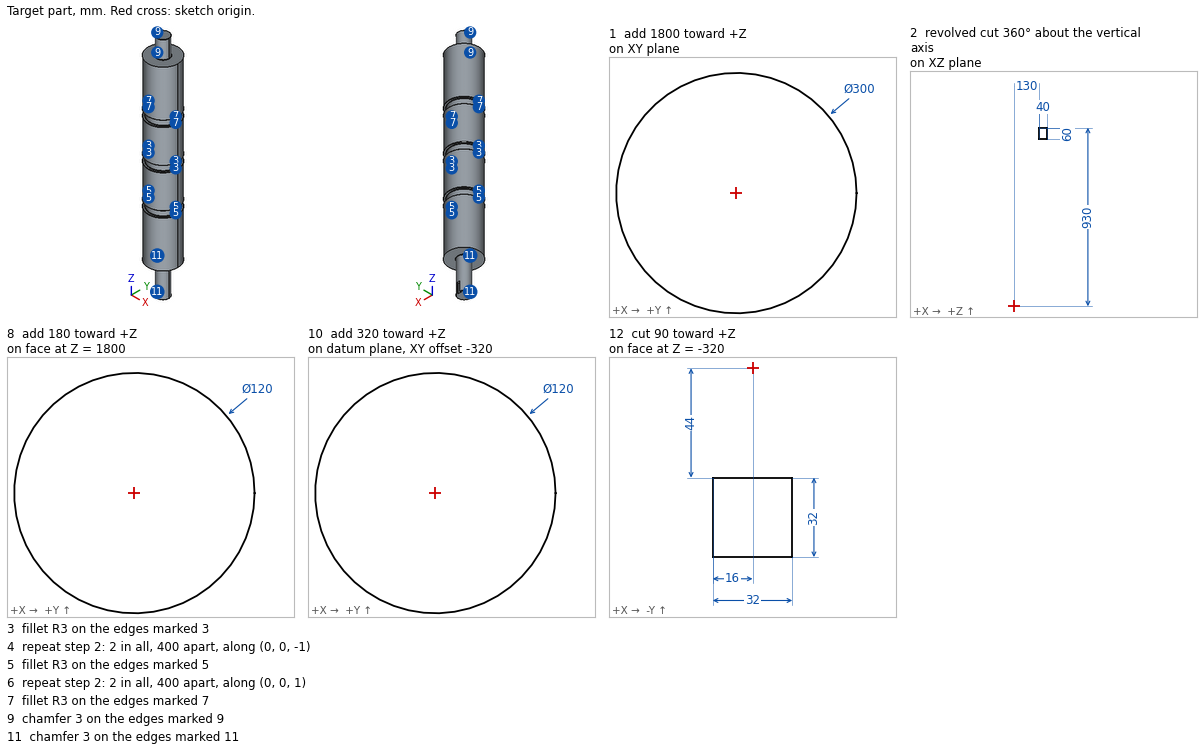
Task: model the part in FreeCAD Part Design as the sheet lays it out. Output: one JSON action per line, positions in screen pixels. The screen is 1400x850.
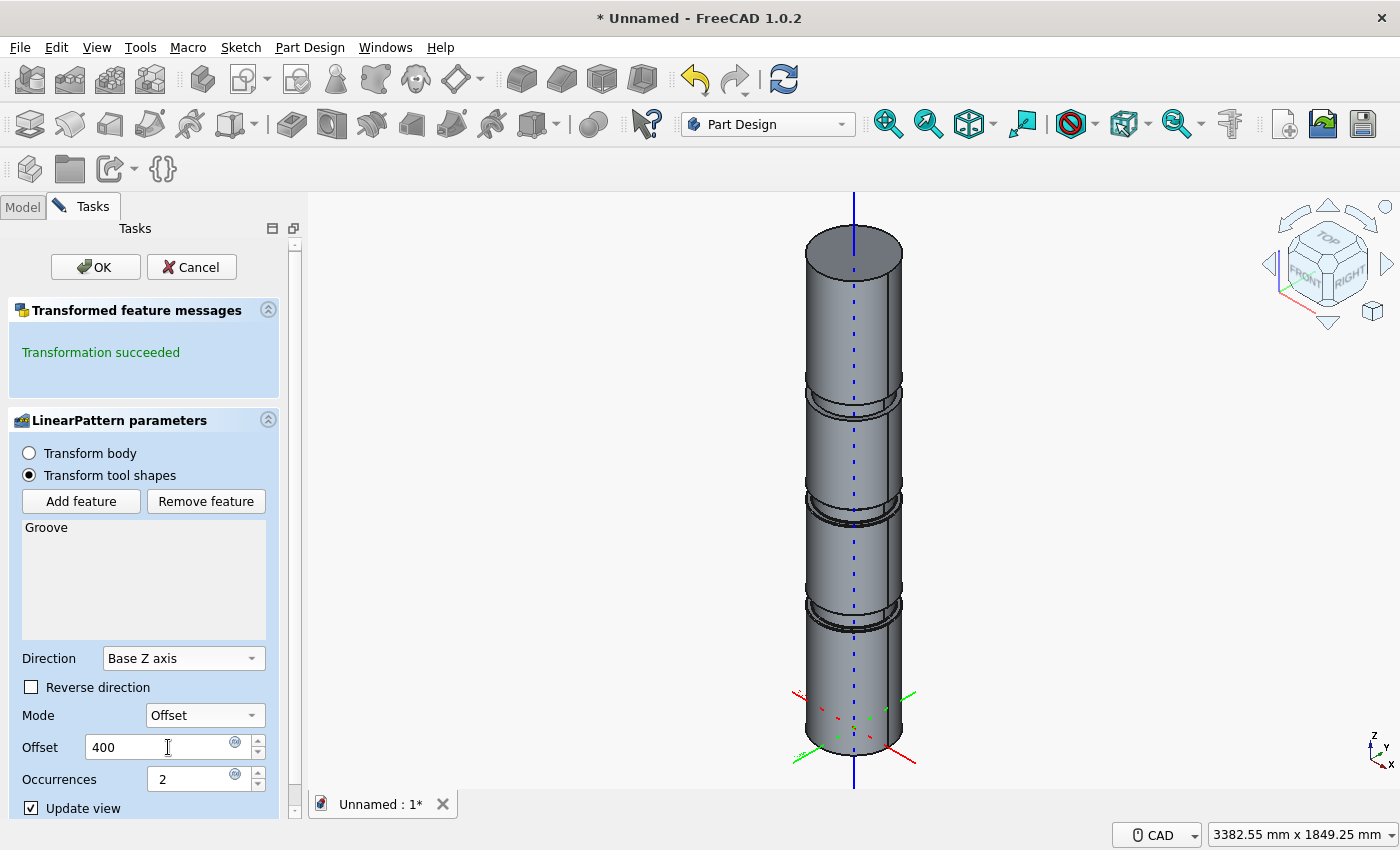
{"action": "triple_click", "coordinate": [198, 779]}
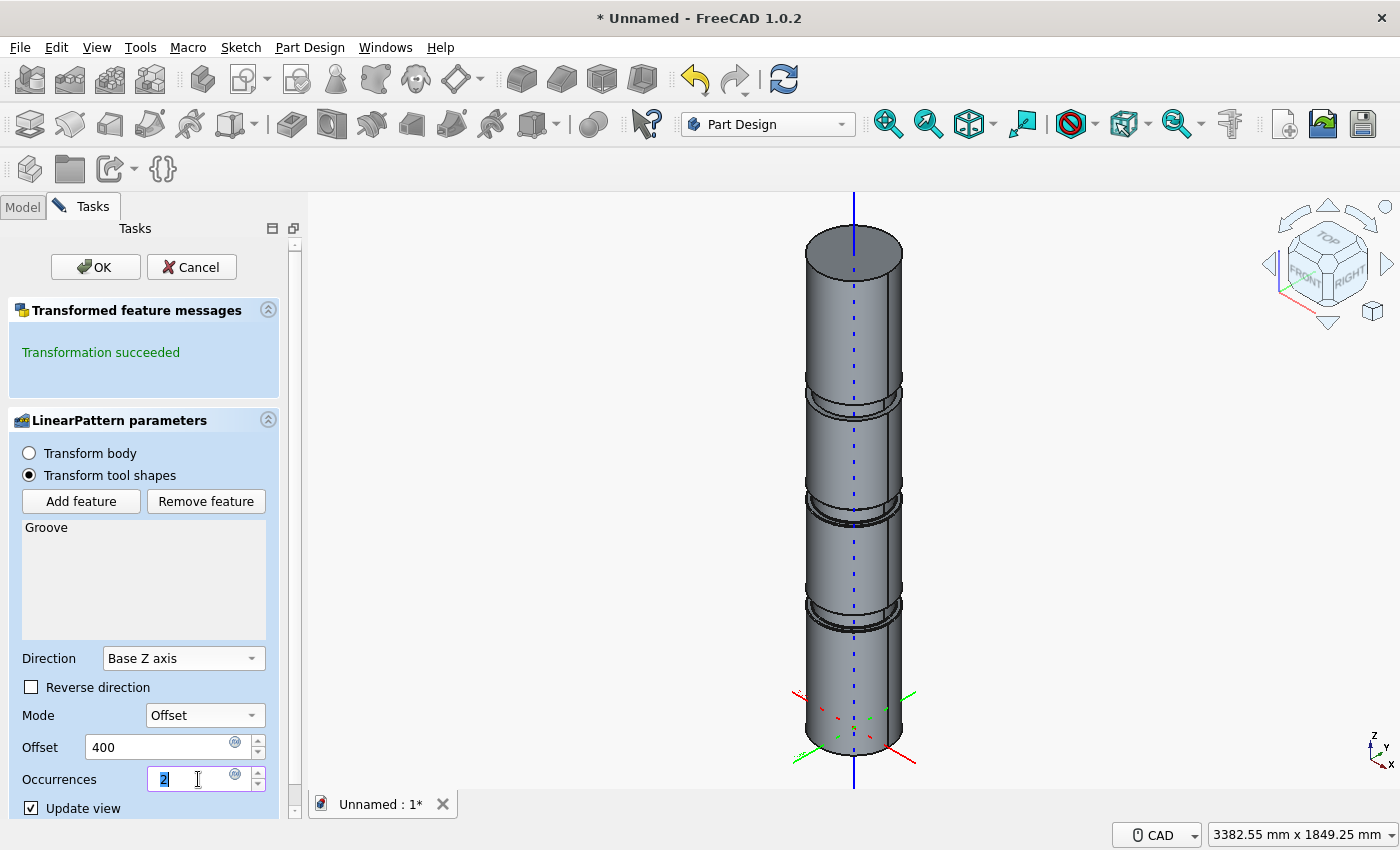
{"action": "type", "text": "2"}
{"action": "key", "text": "Tab"}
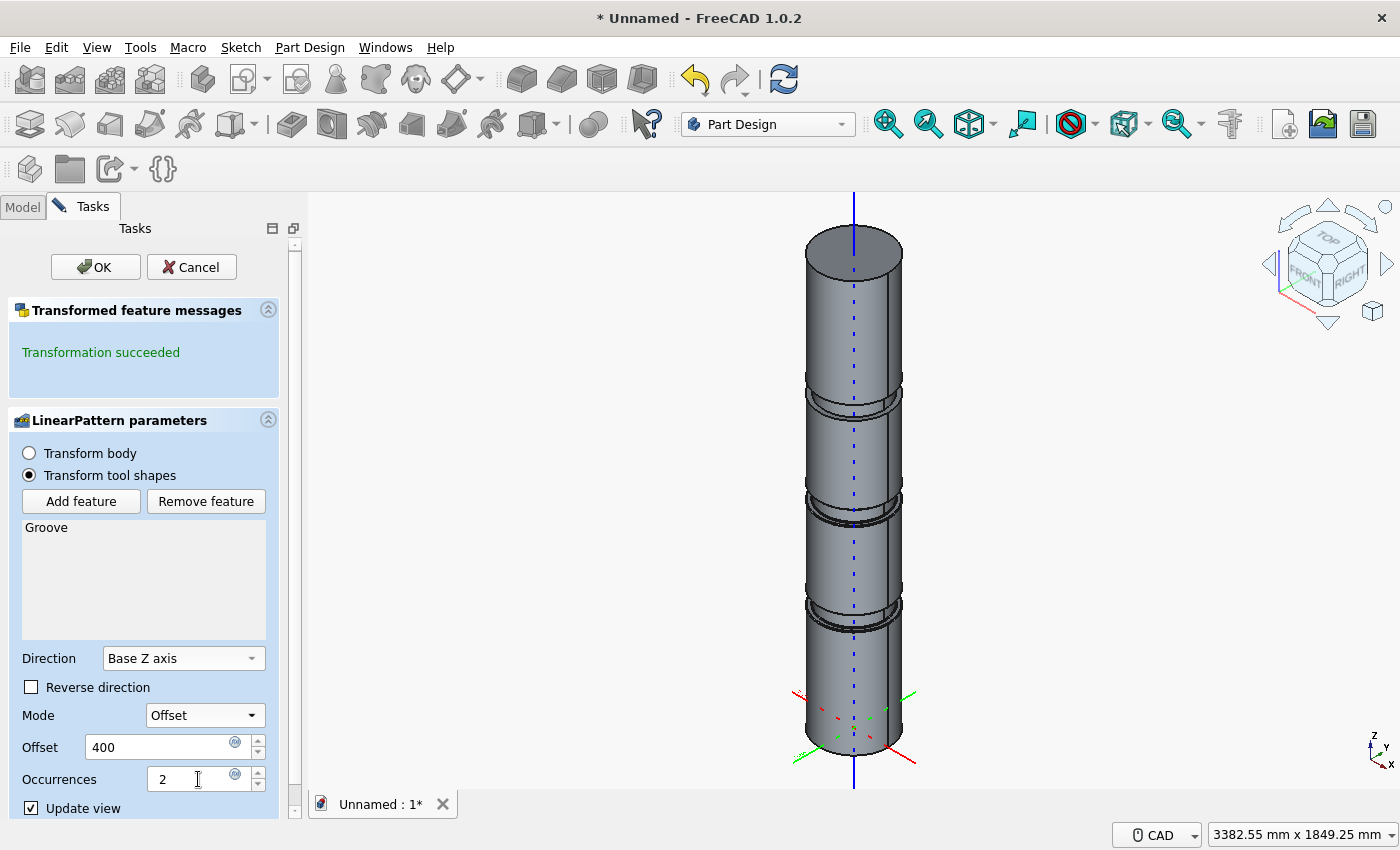
{"action": "left_click", "coordinate": [96, 267]}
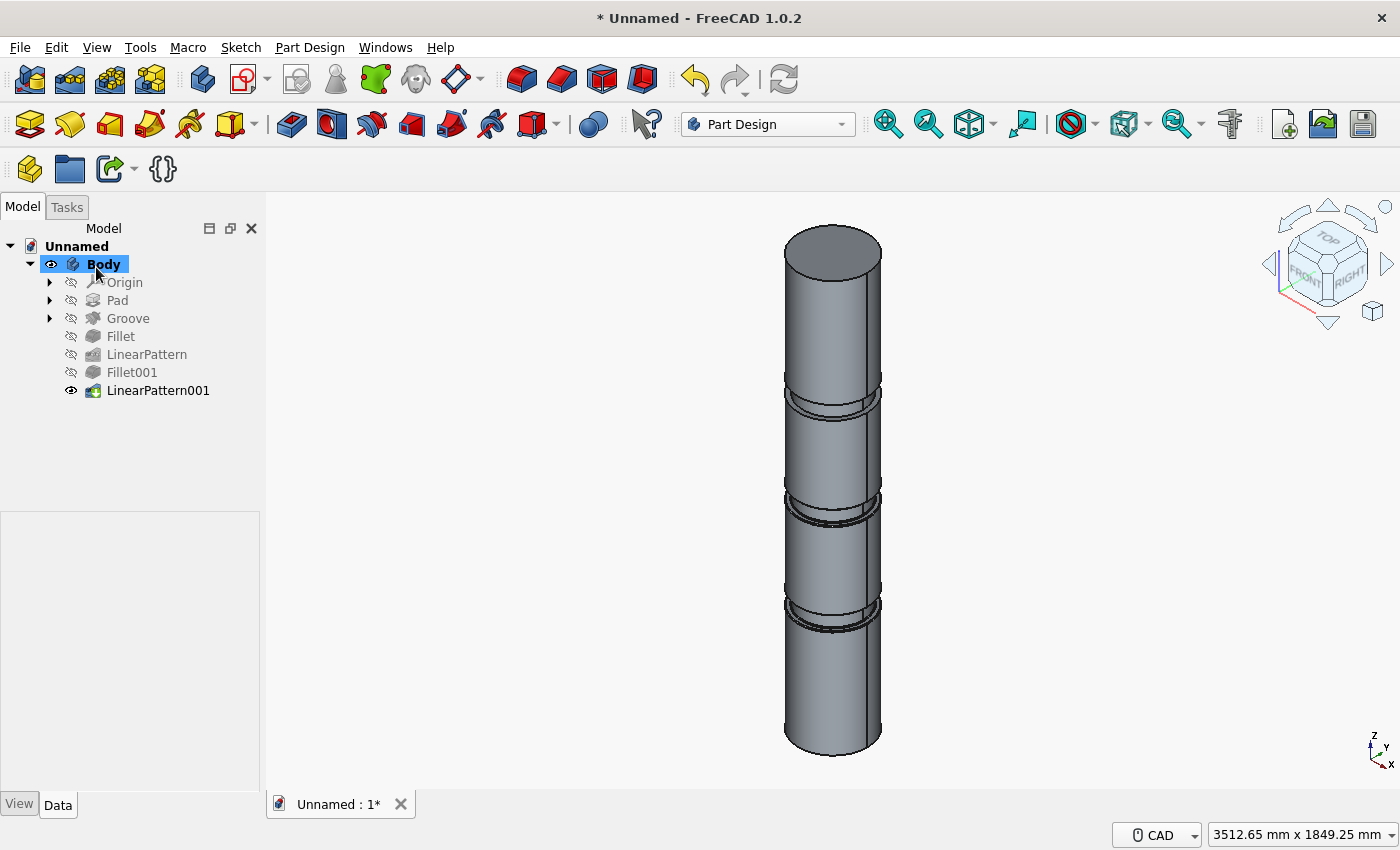
{"action": "left_click", "coordinate": [790, 405]}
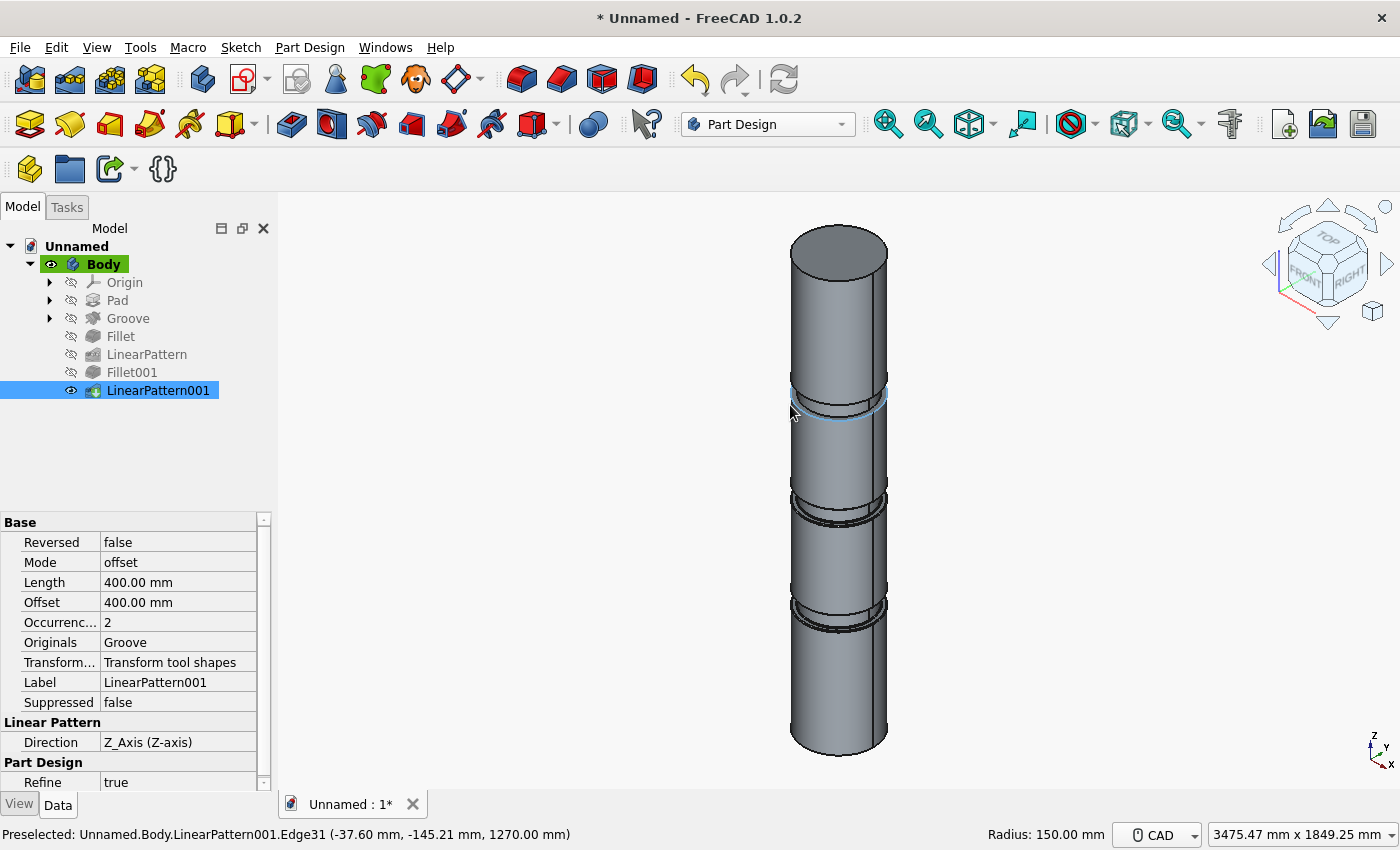
{"action": "key", "text": "2"}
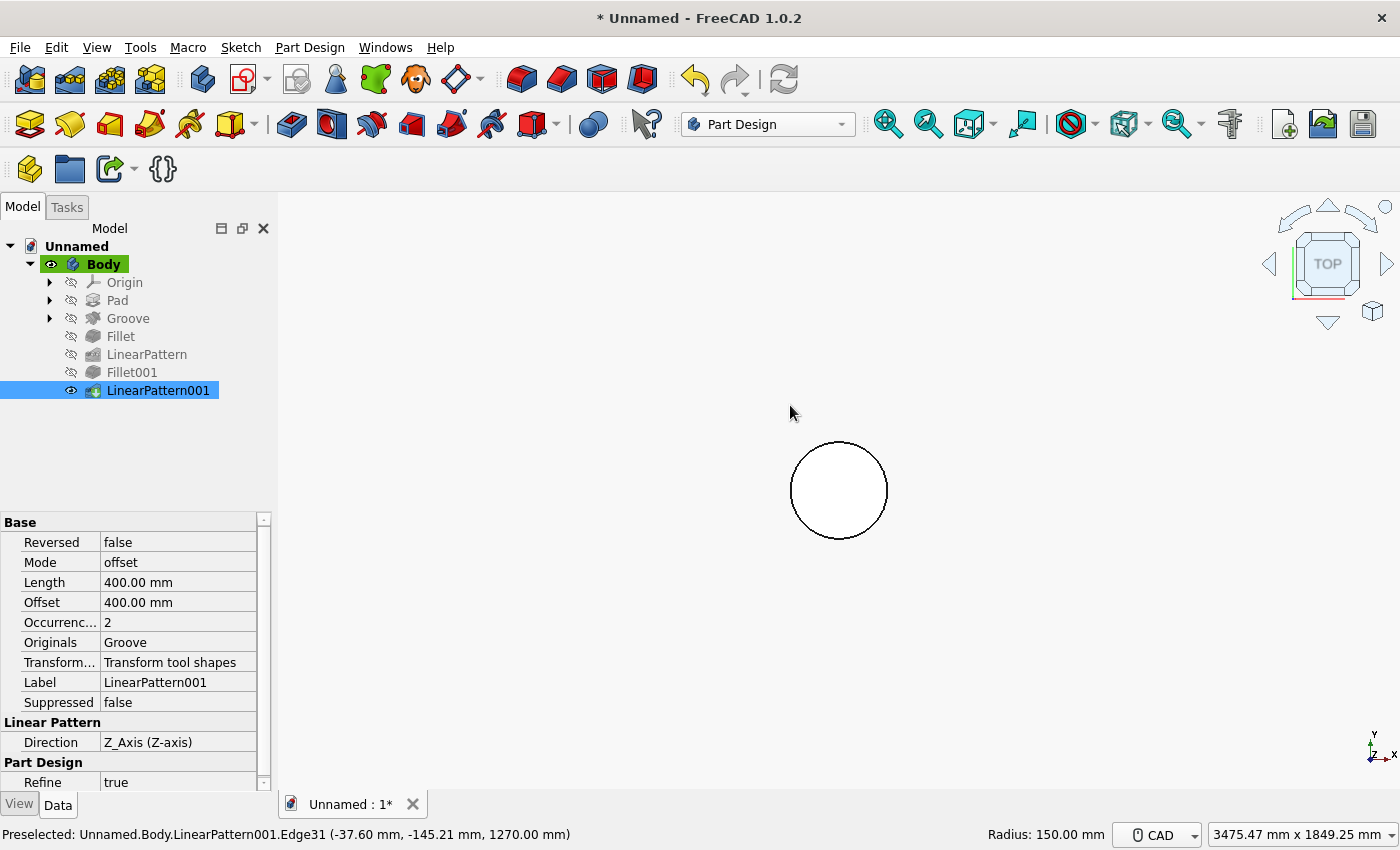
{"action": "left_click", "coordinate": [890, 124]}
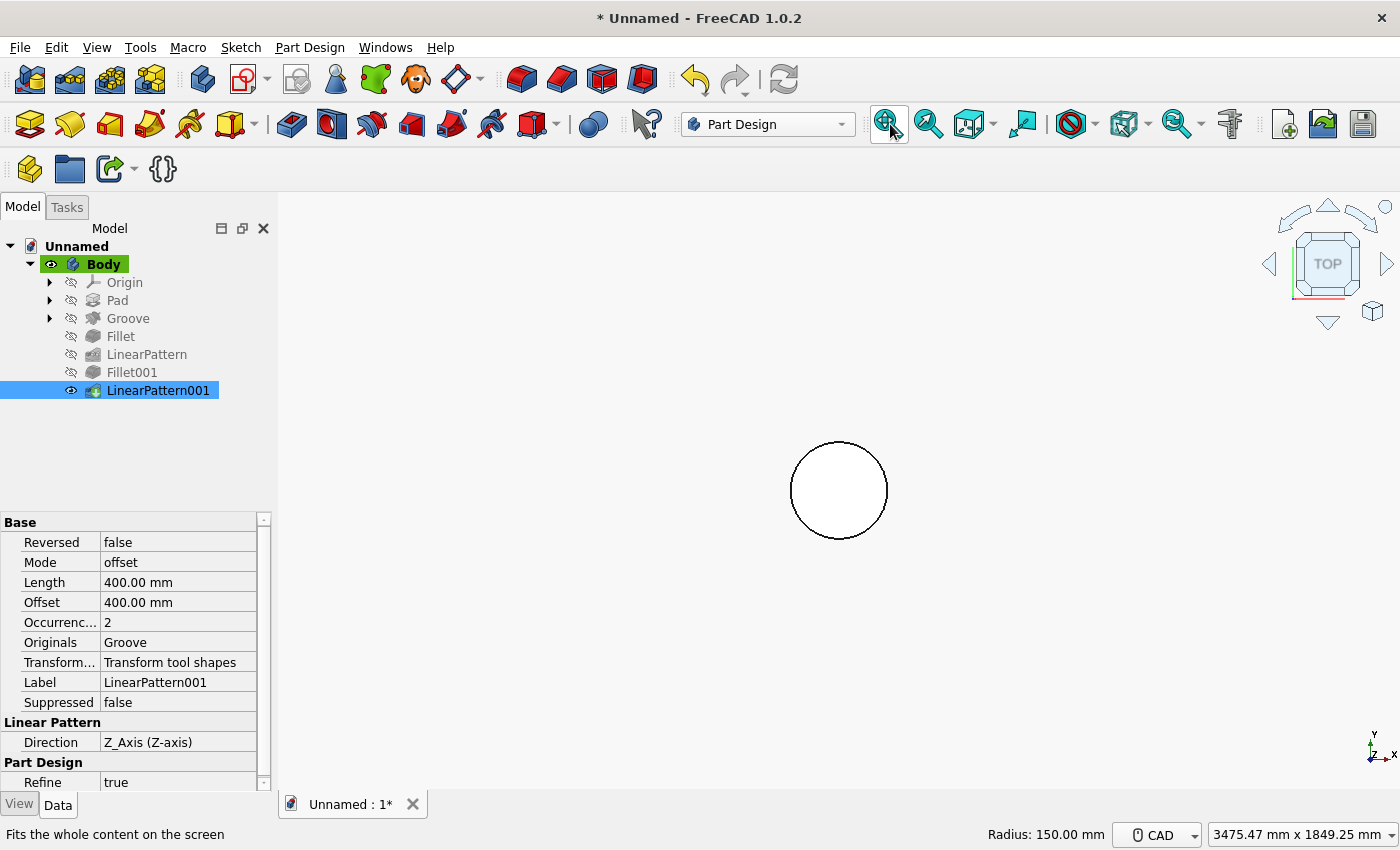
{"action": "key", "text": "0"}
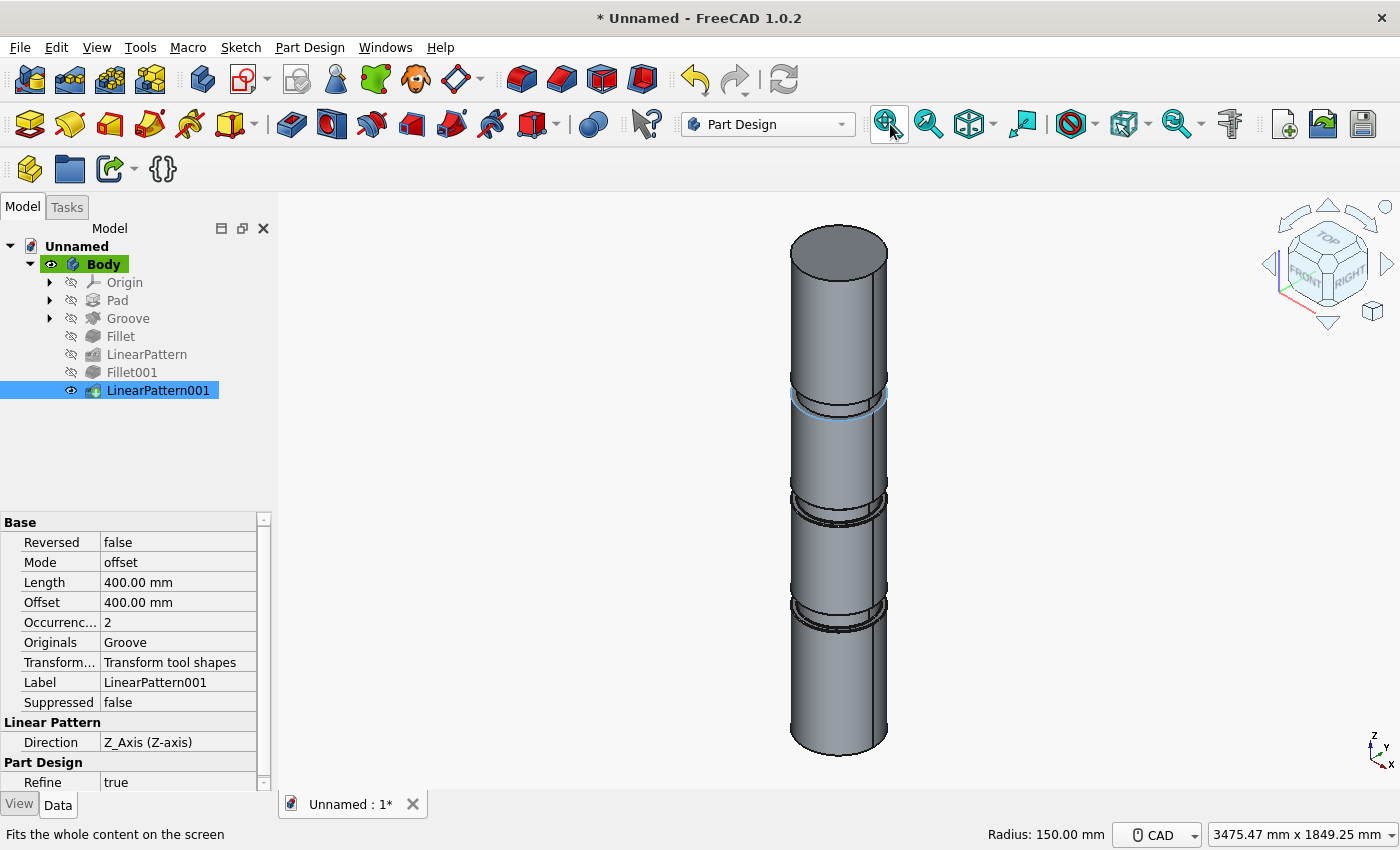
{"action": "key", "text": "1"}